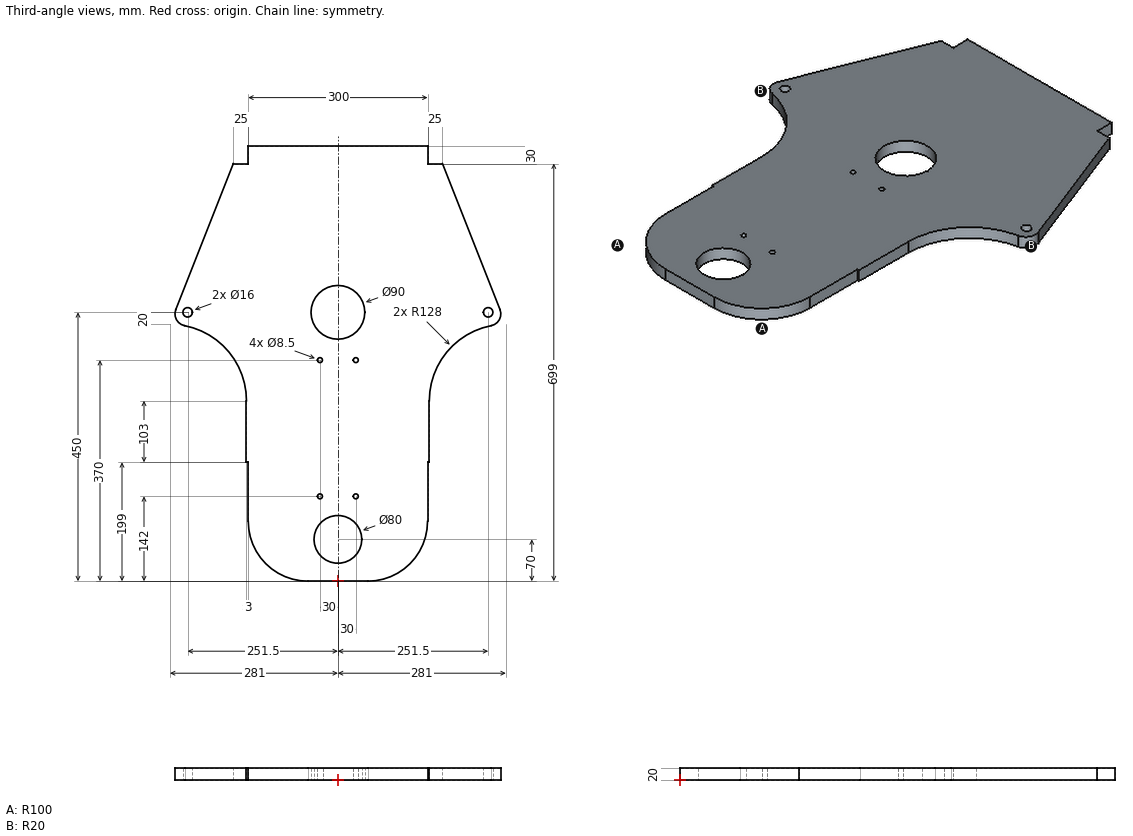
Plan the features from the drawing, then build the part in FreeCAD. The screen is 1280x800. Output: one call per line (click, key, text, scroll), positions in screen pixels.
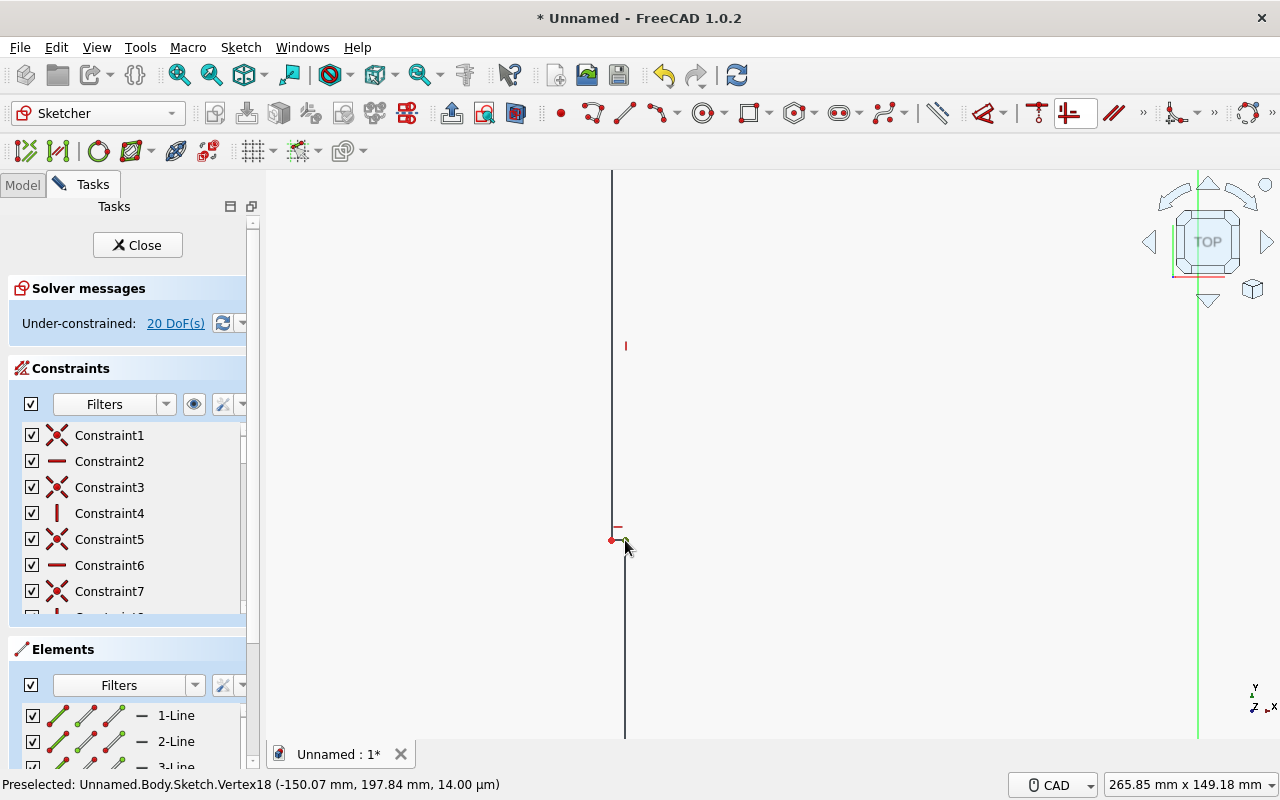
scroll(627, 541, down, 10)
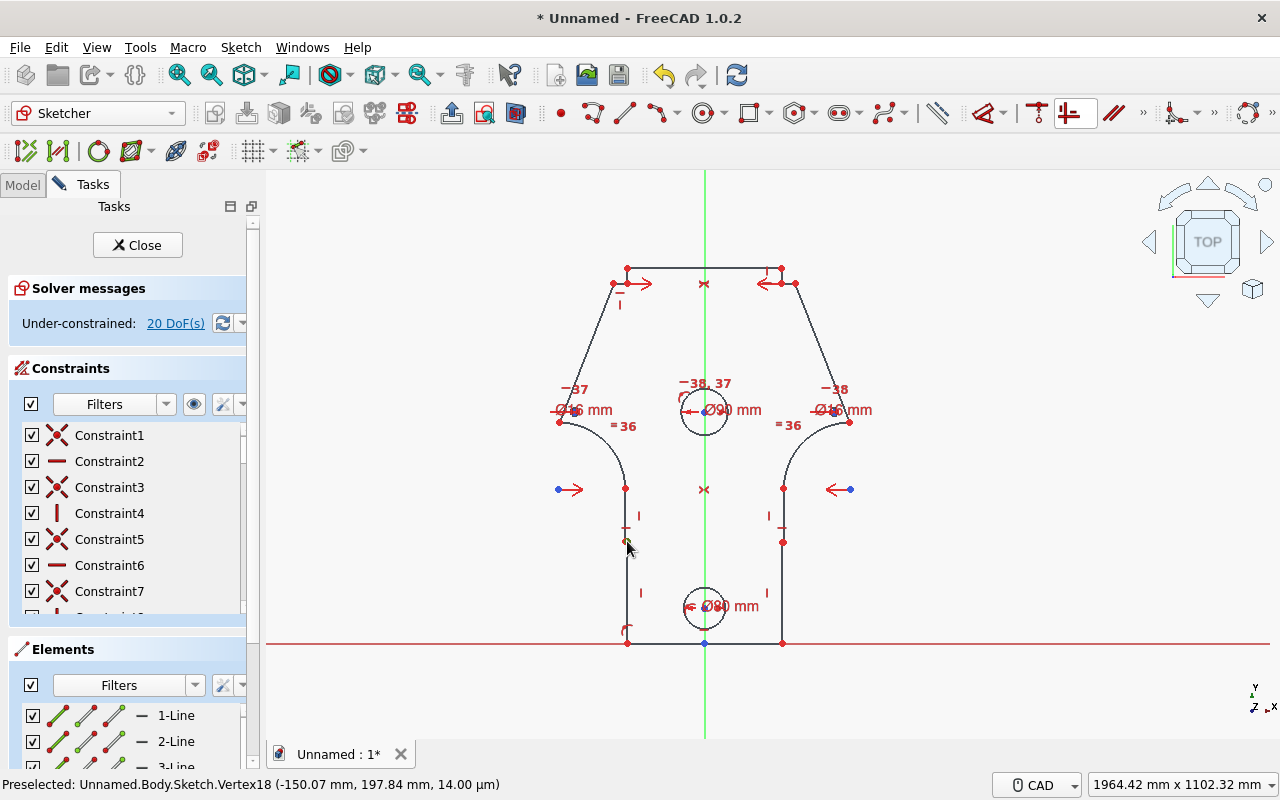
scroll(782, 542, up, 11)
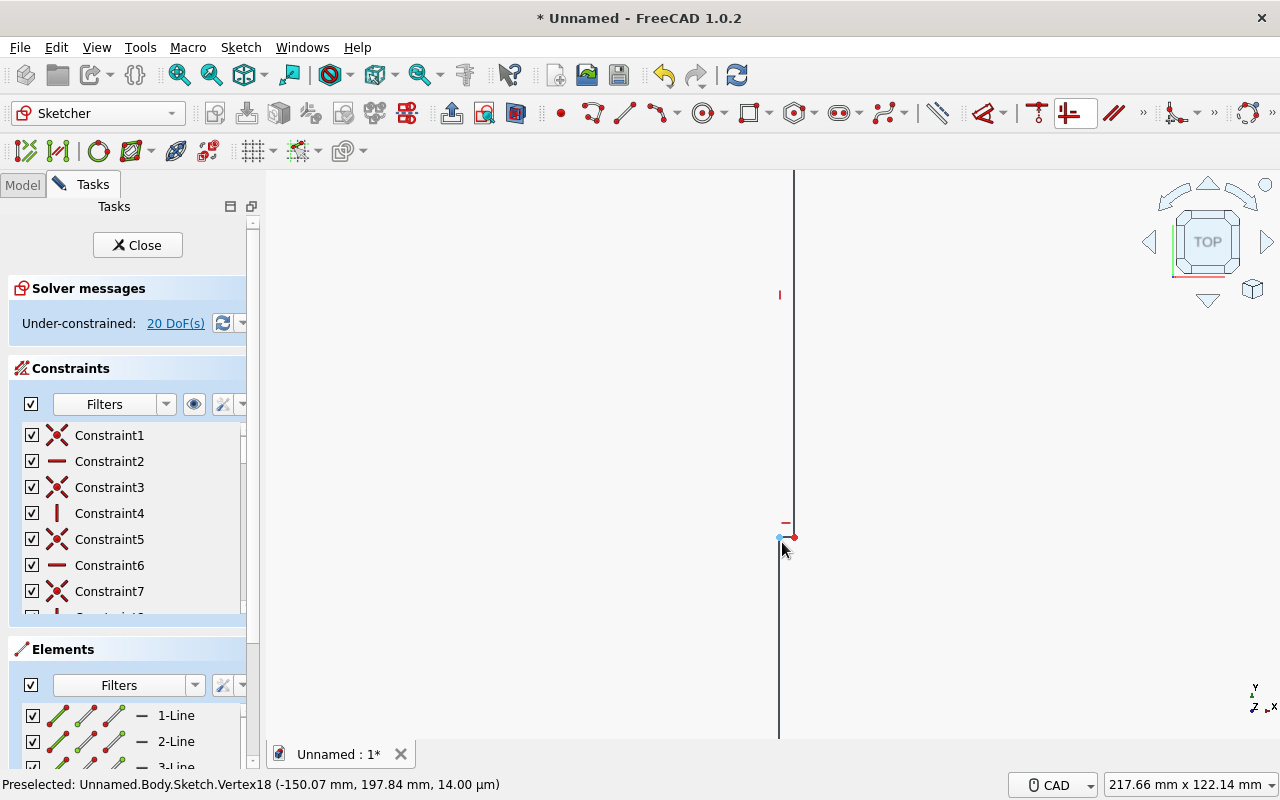
click(779, 537)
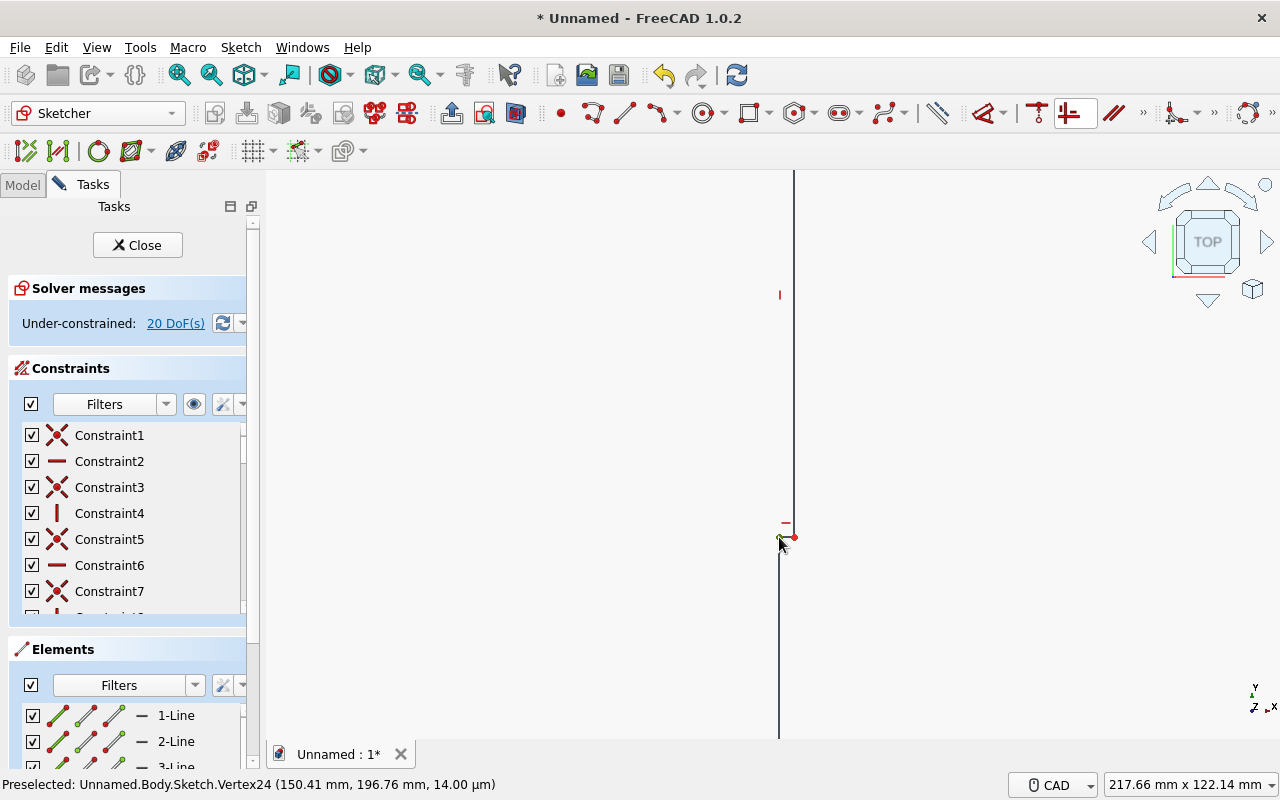
scroll(782, 542, down, 11)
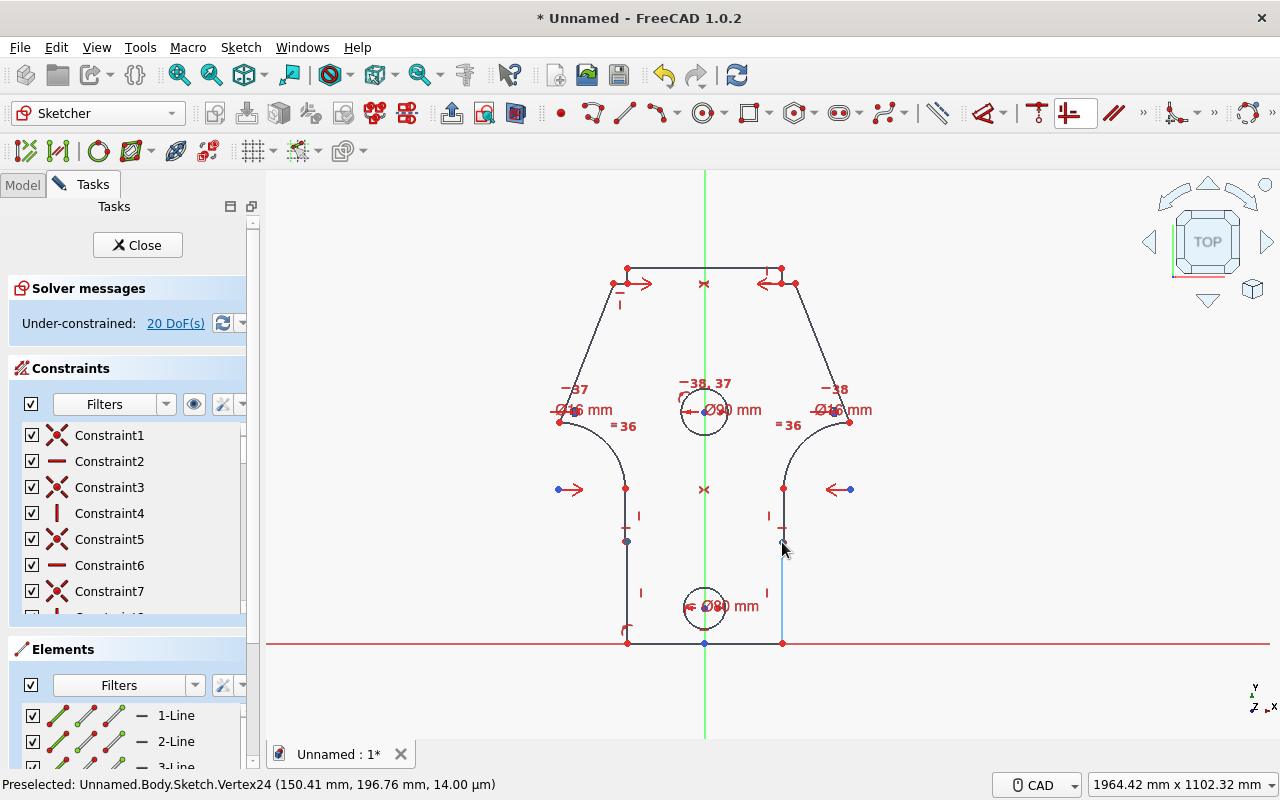
click(705, 674)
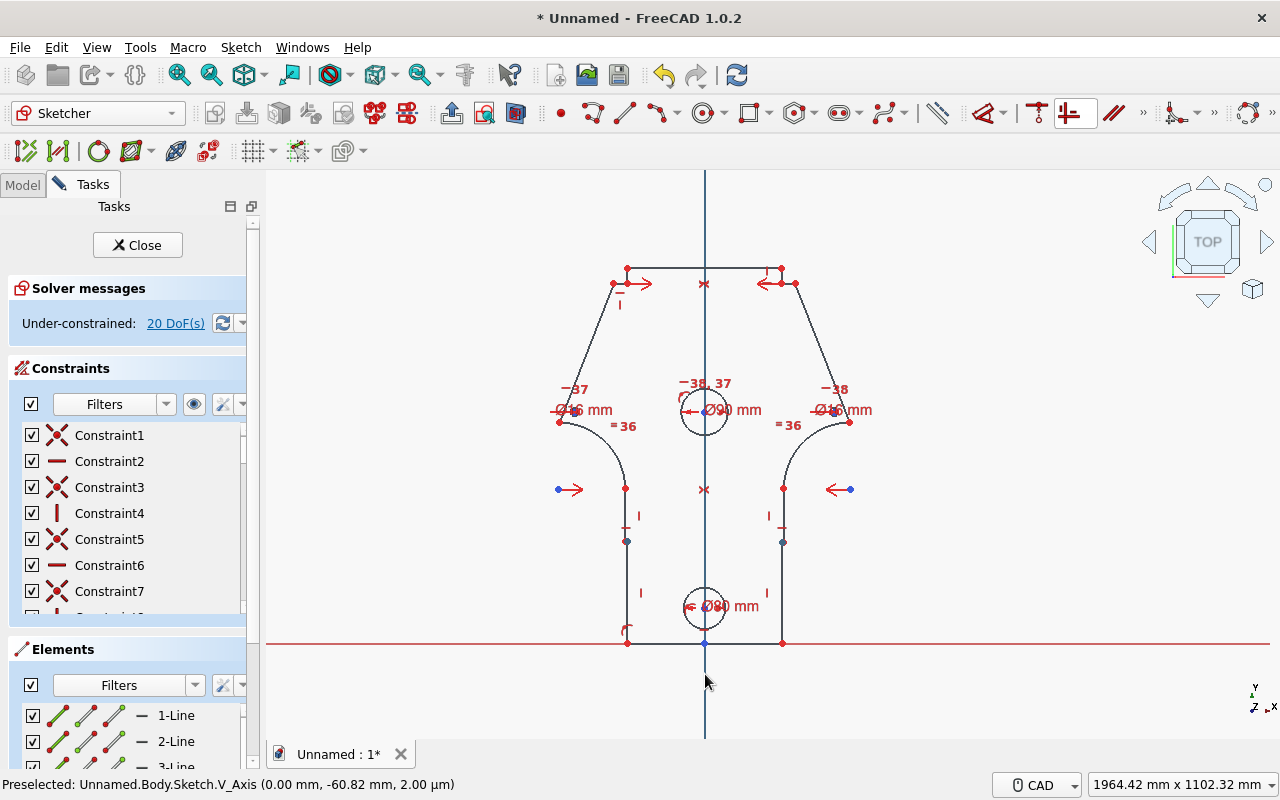
key(s)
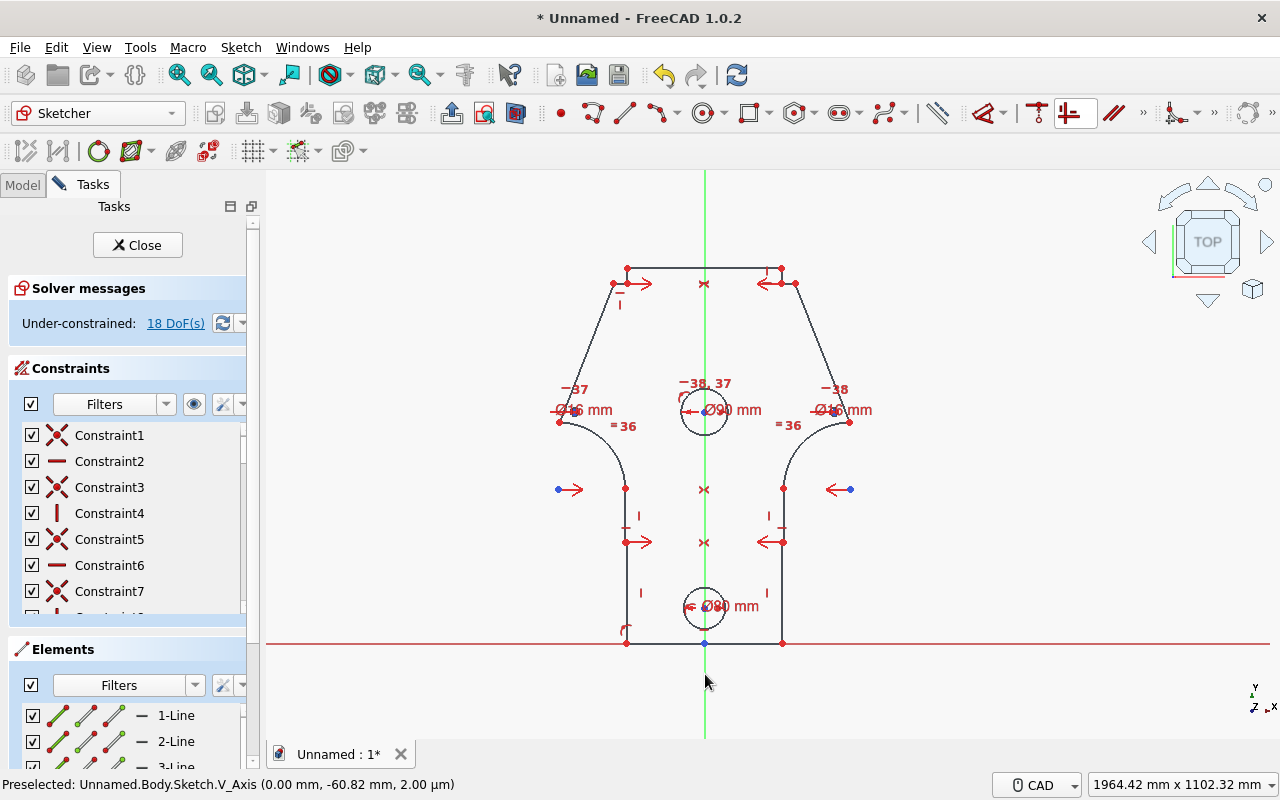
click(984, 114)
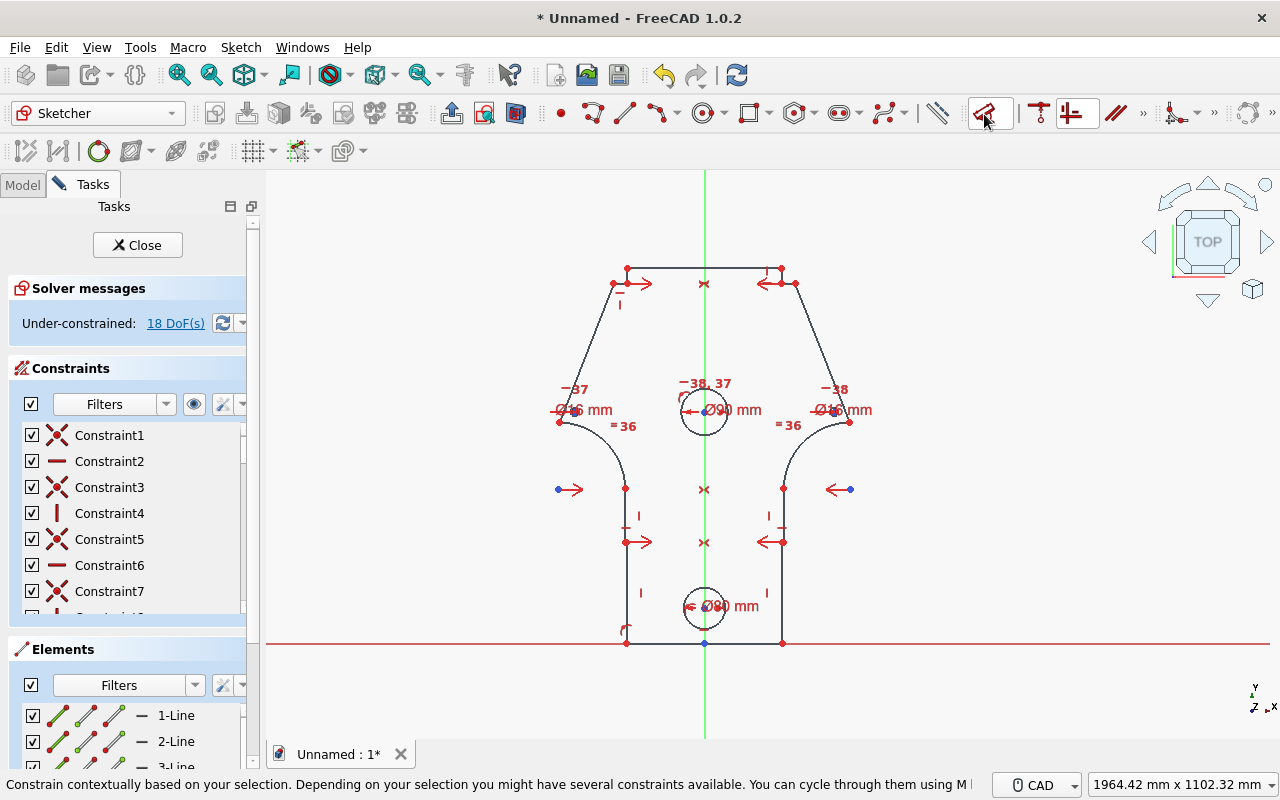
click(618, 459)
click(646, 444)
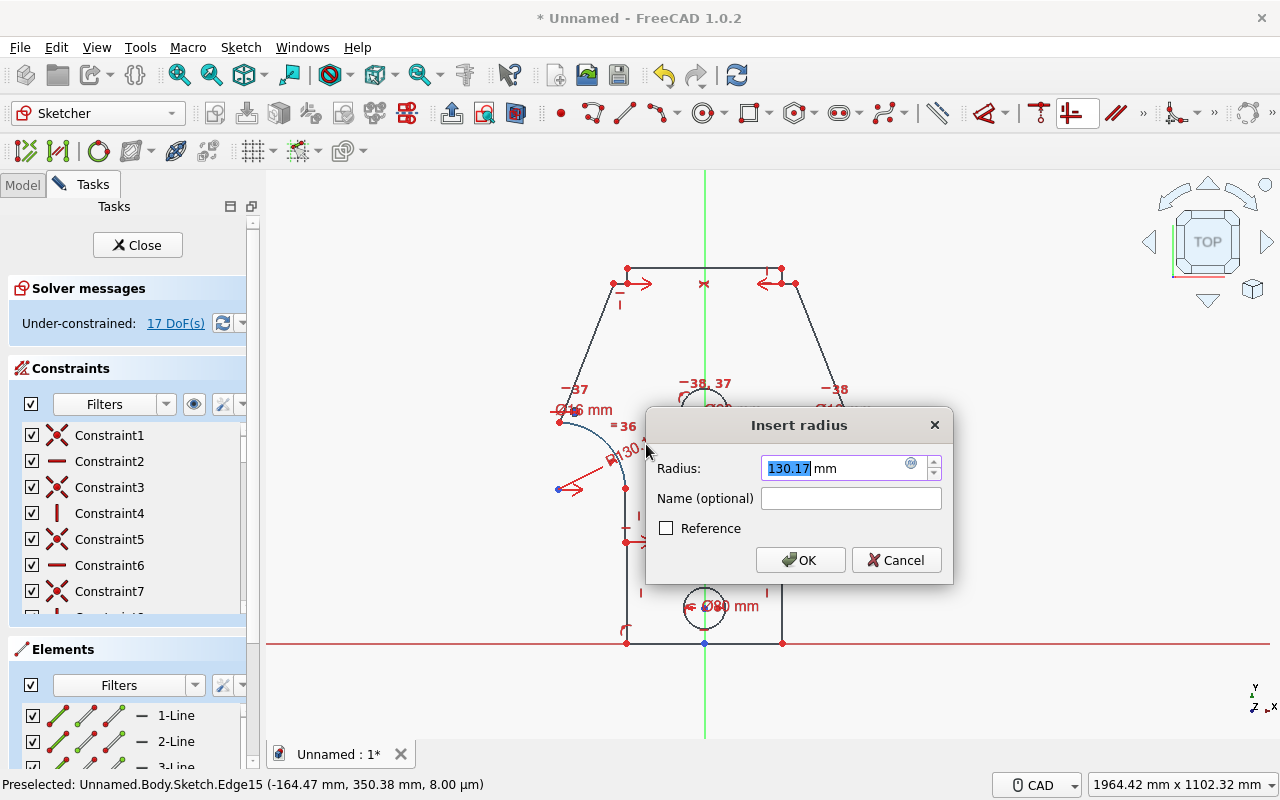
text(128)
key(Return)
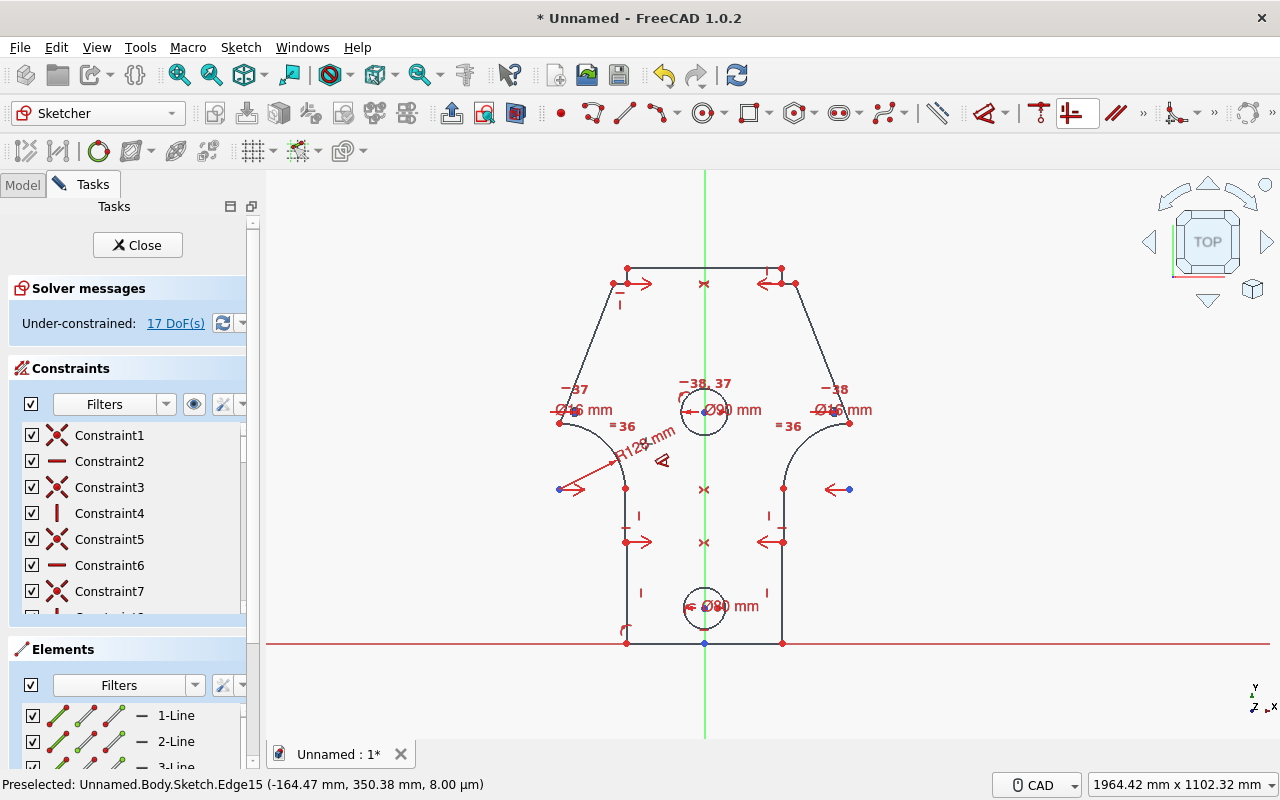
scroll(626, 542, up, 17)